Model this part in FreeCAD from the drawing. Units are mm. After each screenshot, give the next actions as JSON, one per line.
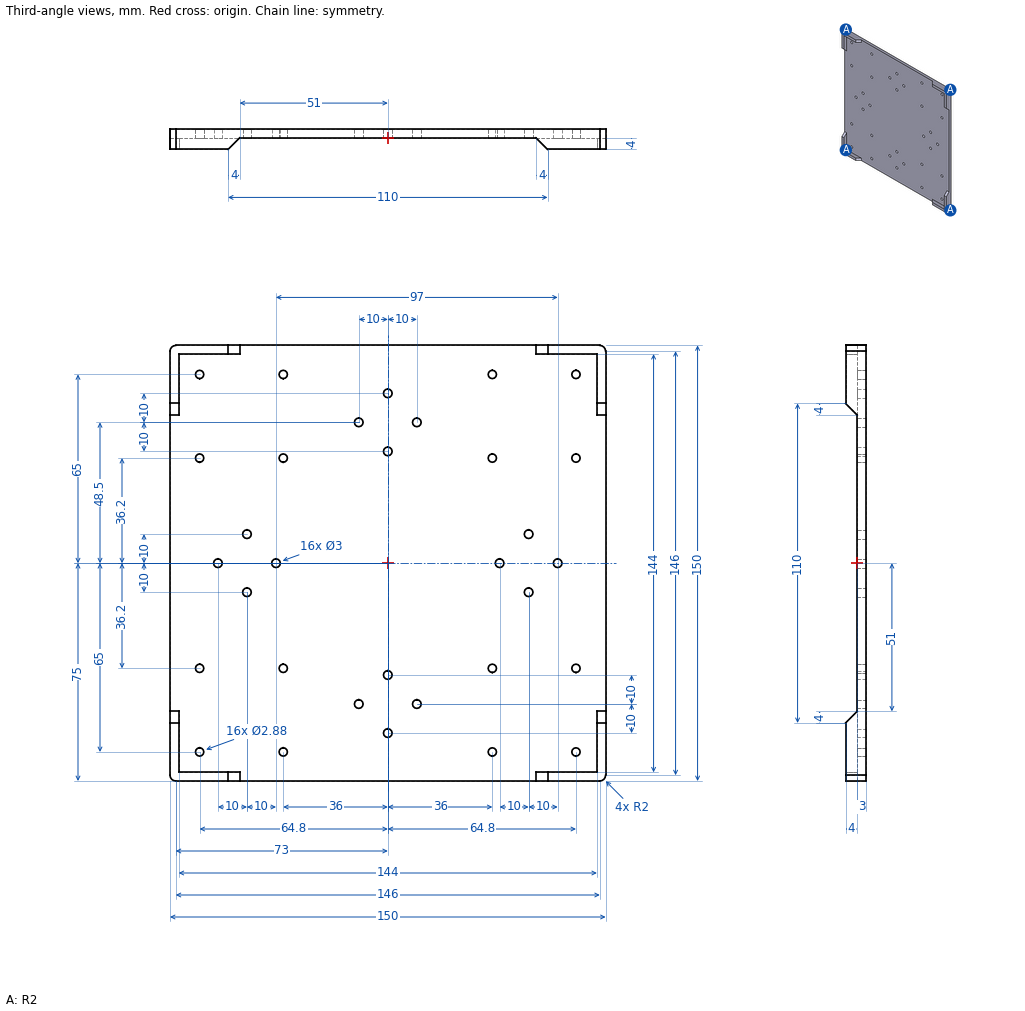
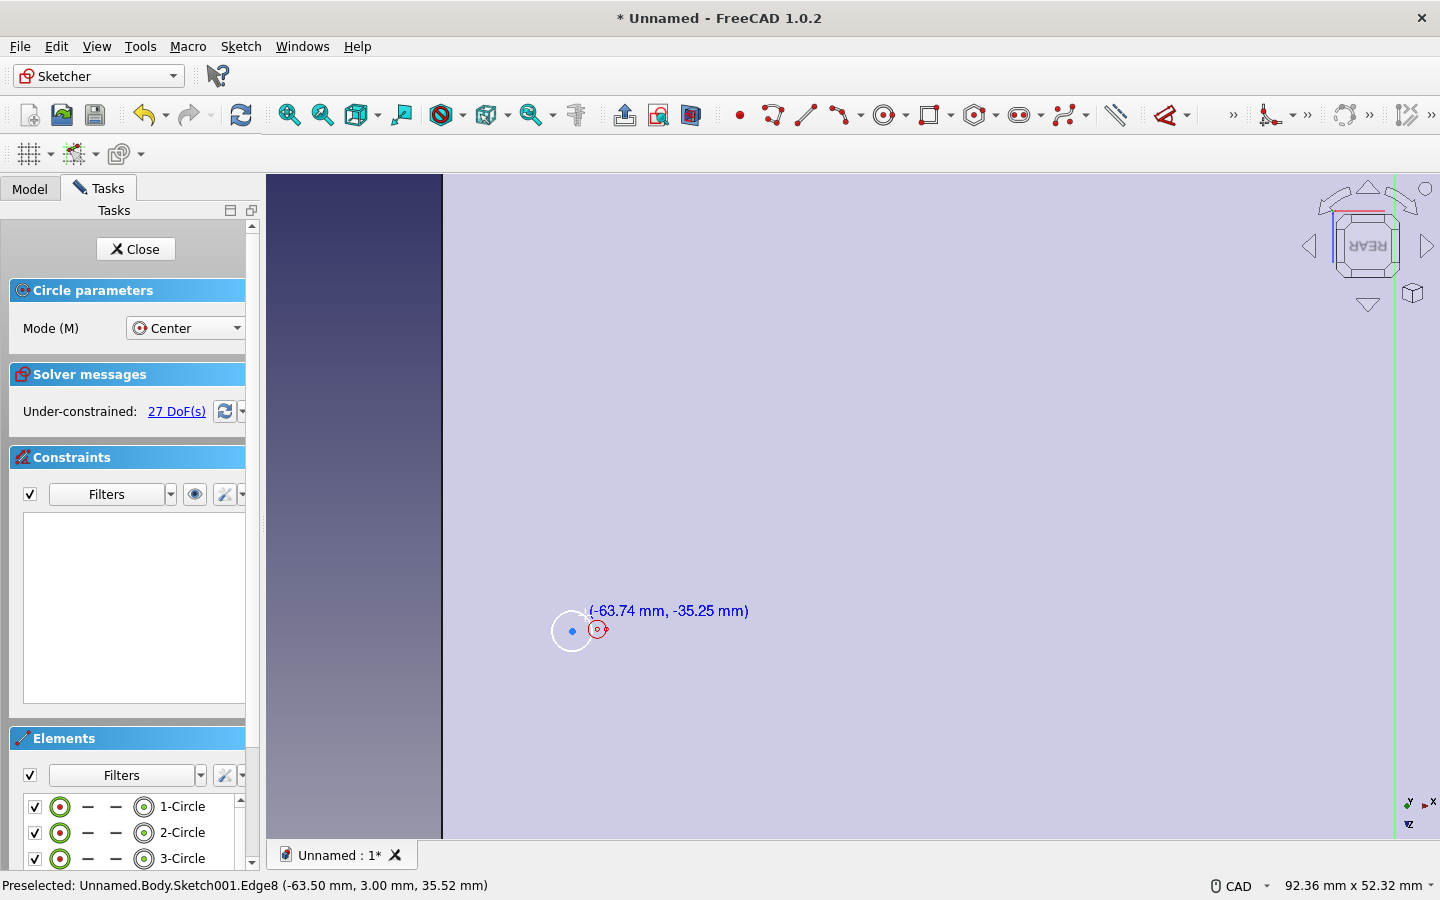
{"action": "scroll", "coordinate": [585, 617], "scroll_direction": "down", "scroll_amount": 7}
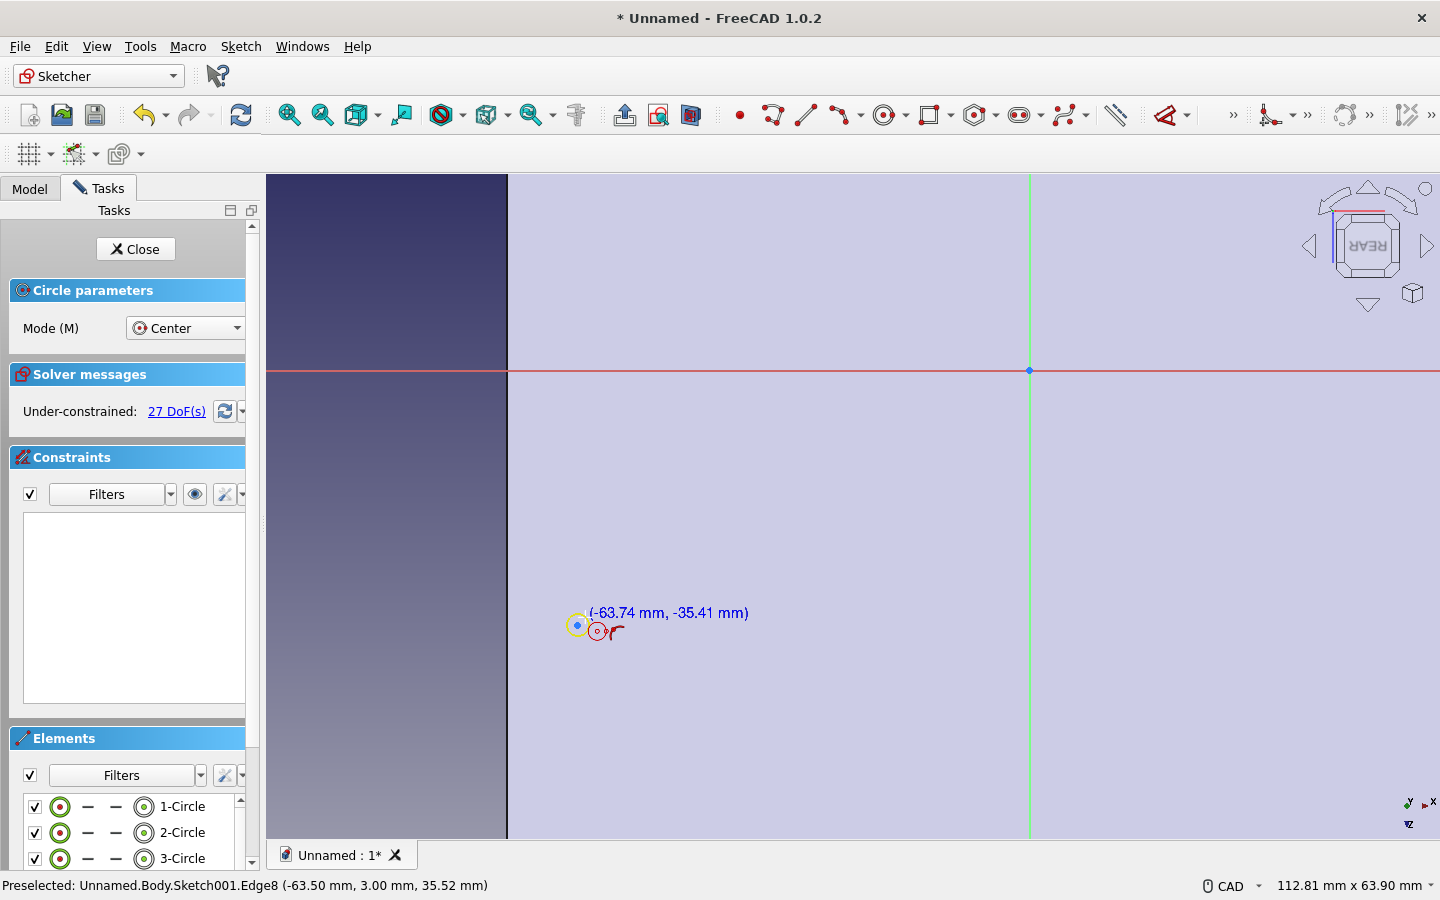
{"action": "scroll", "coordinate": [582, 711], "scroll_direction": "up", "scroll_amount": 9}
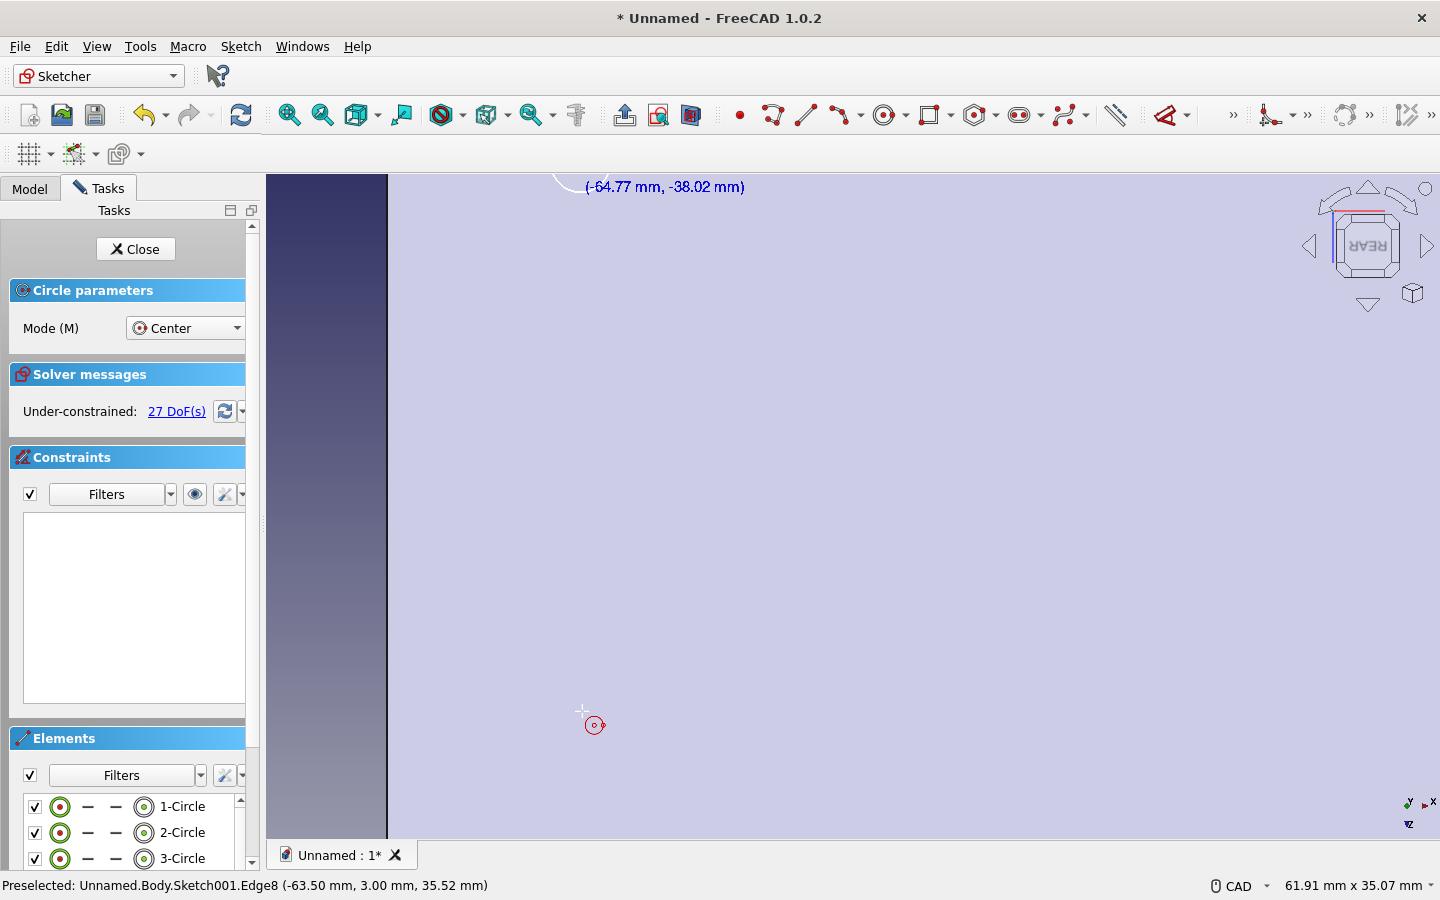
{"action": "scroll", "coordinate": [582, 711], "scroll_direction": "down", "scroll_amount": 9}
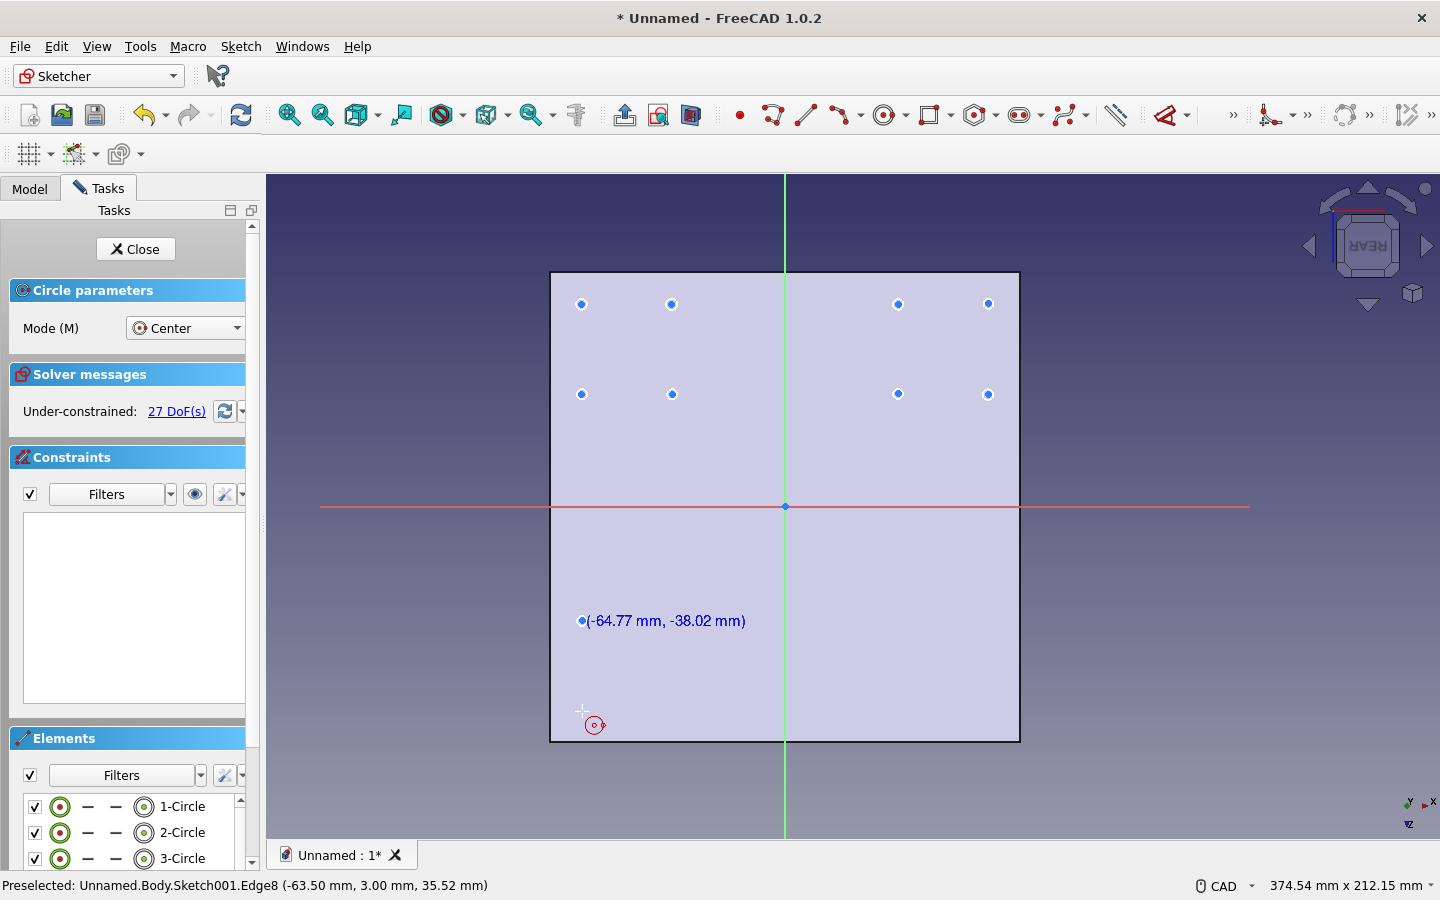
{"action": "left_click", "coordinate": [582, 711]}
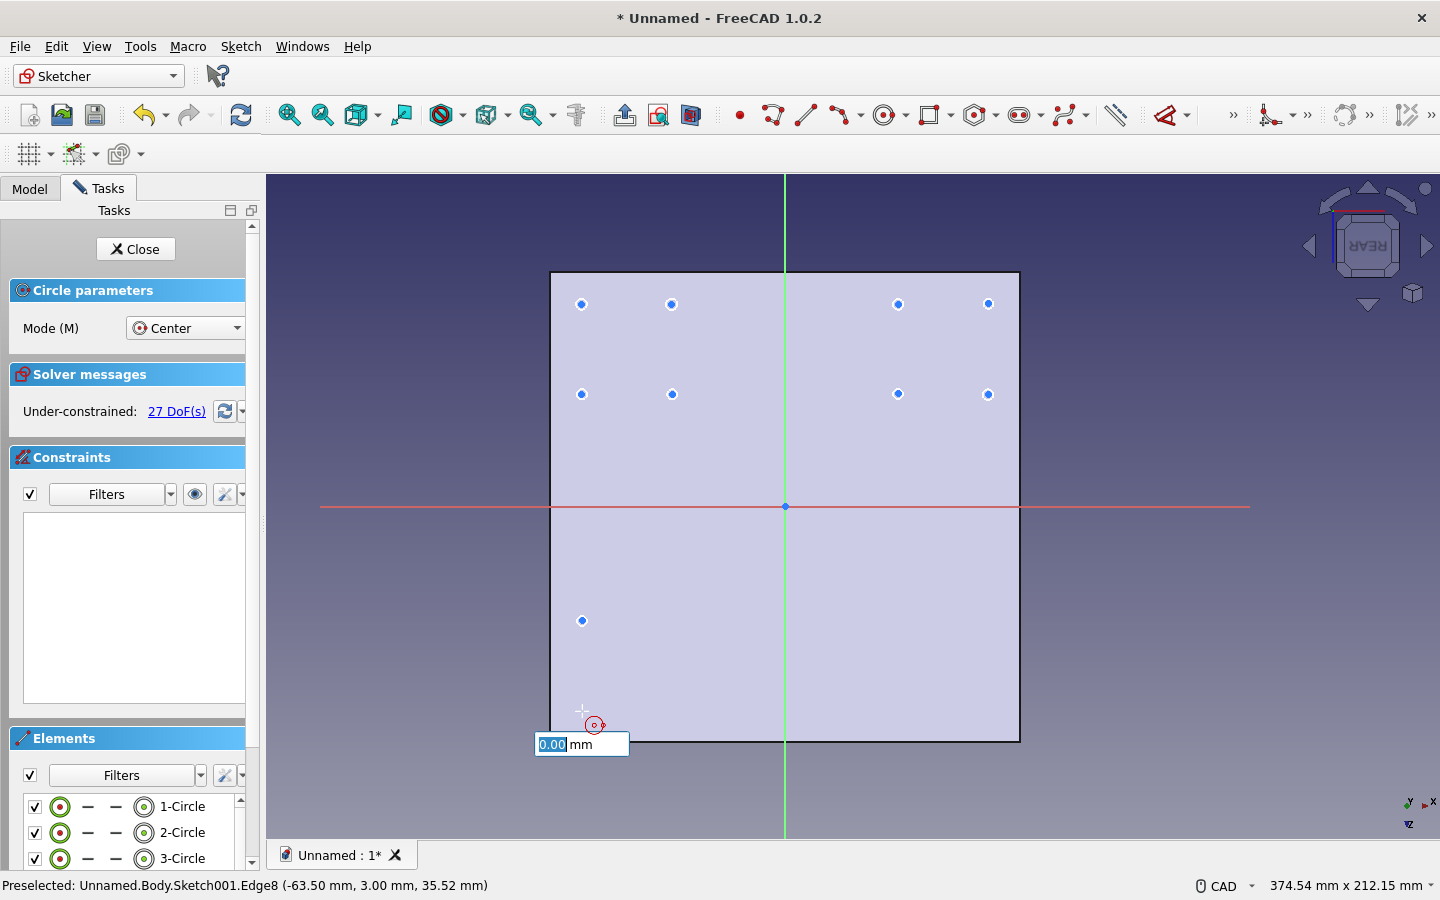
{"action": "scroll", "coordinate": [585, 707], "scroll_direction": "up", "scroll_amount": 7}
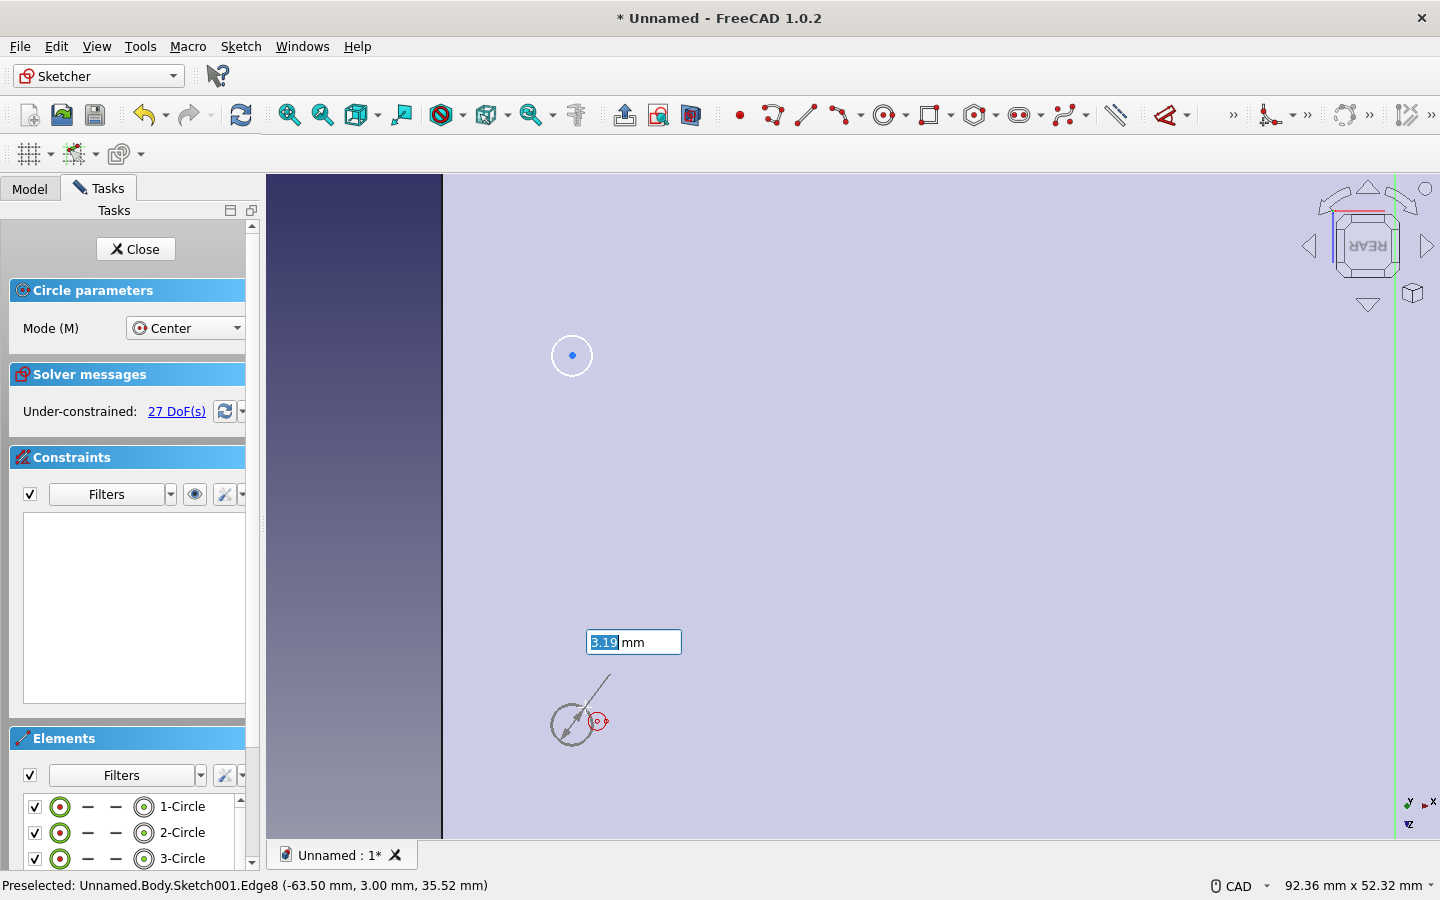
{"action": "left_click", "coordinate": [585, 706]}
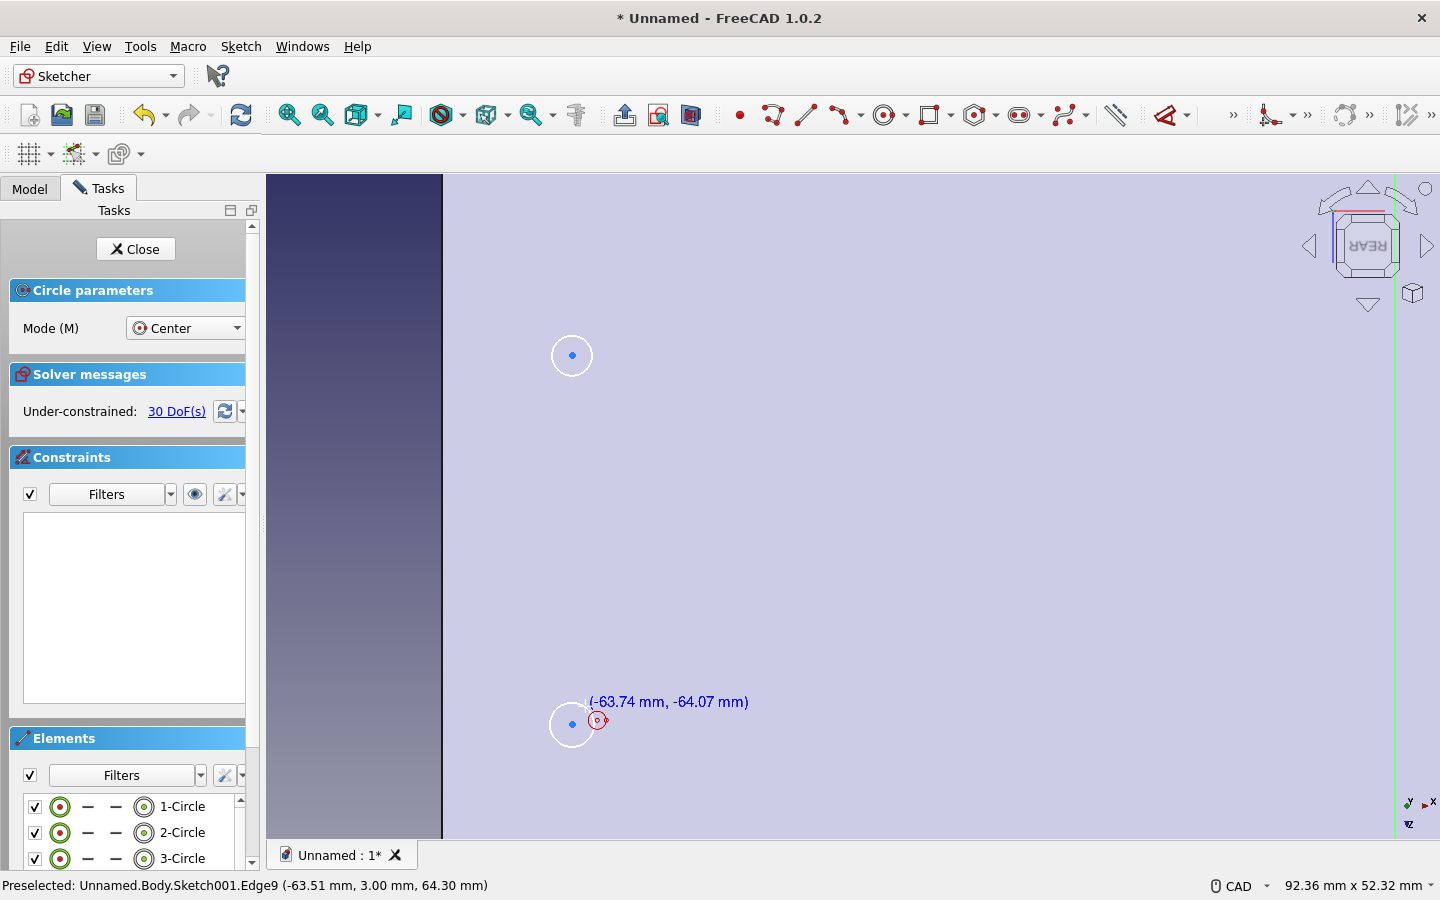
{"action": "scroll", "coordinate": [938, 719], "scroll_direction": "up", "scroll_amount": 2}